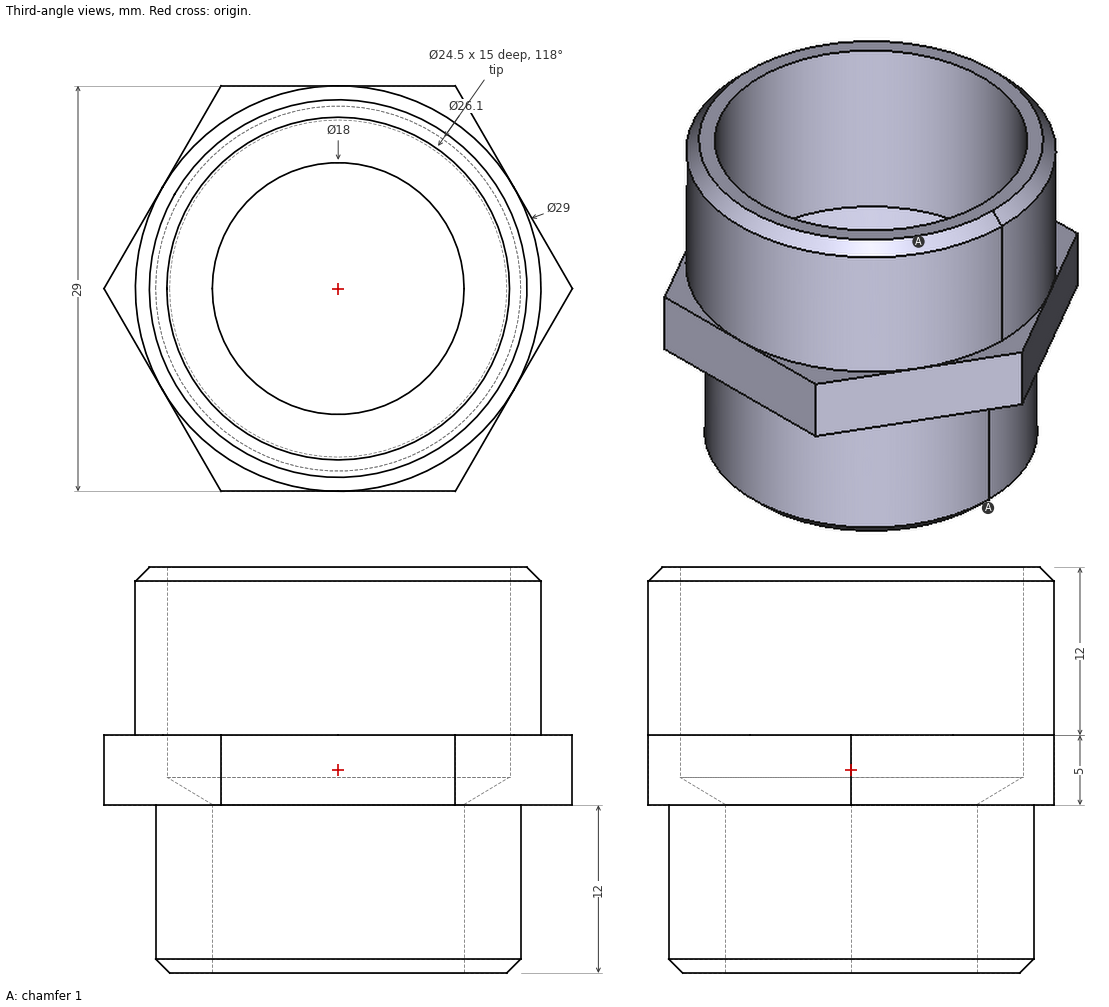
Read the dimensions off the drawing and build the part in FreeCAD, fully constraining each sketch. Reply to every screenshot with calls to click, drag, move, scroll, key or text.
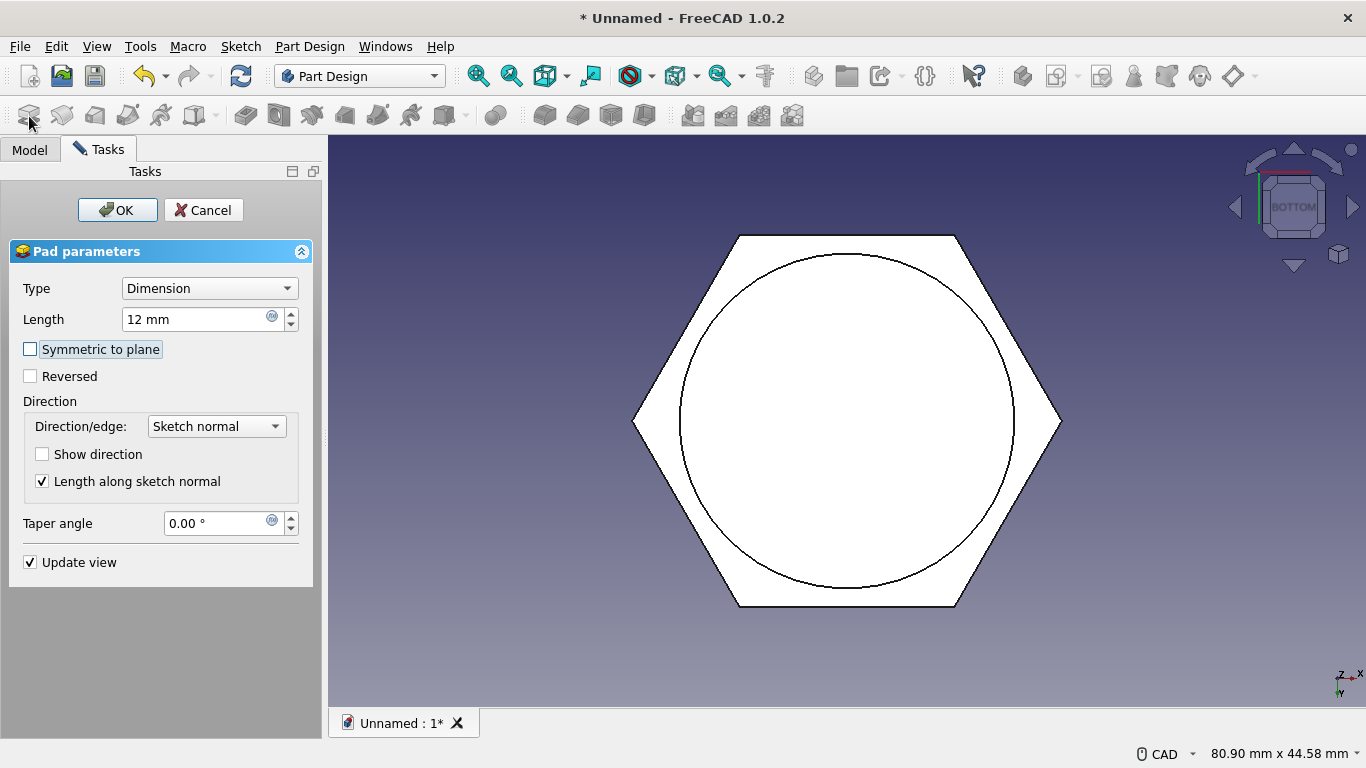
click(118, 210)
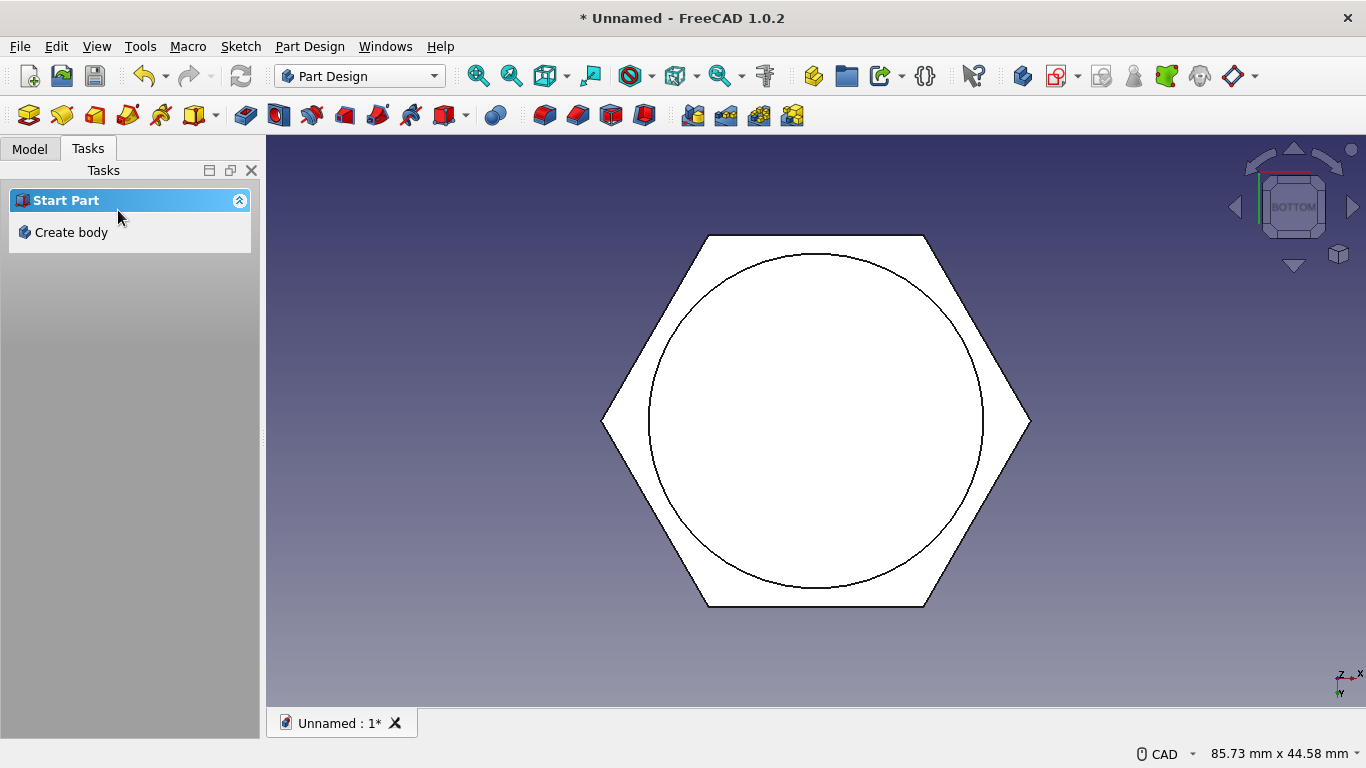
click(816, 420)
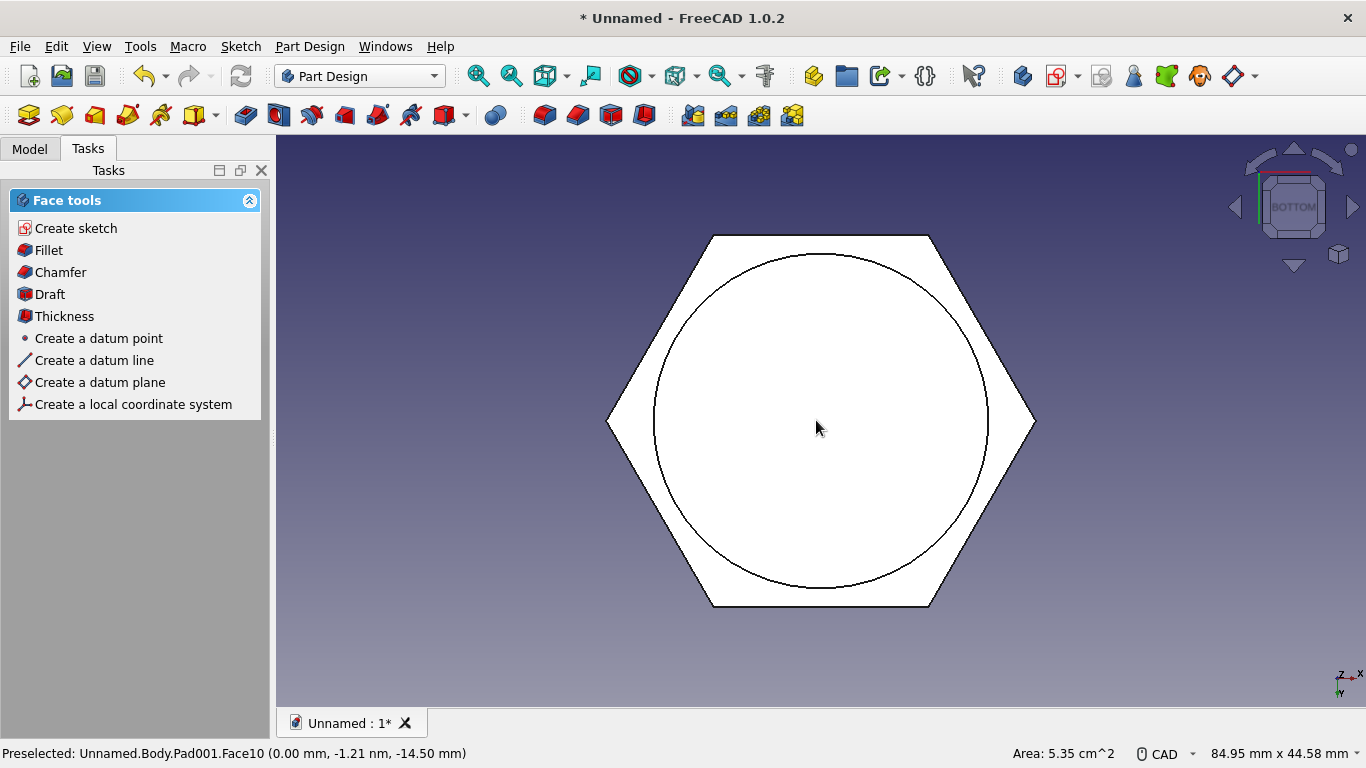
click(1056, 76)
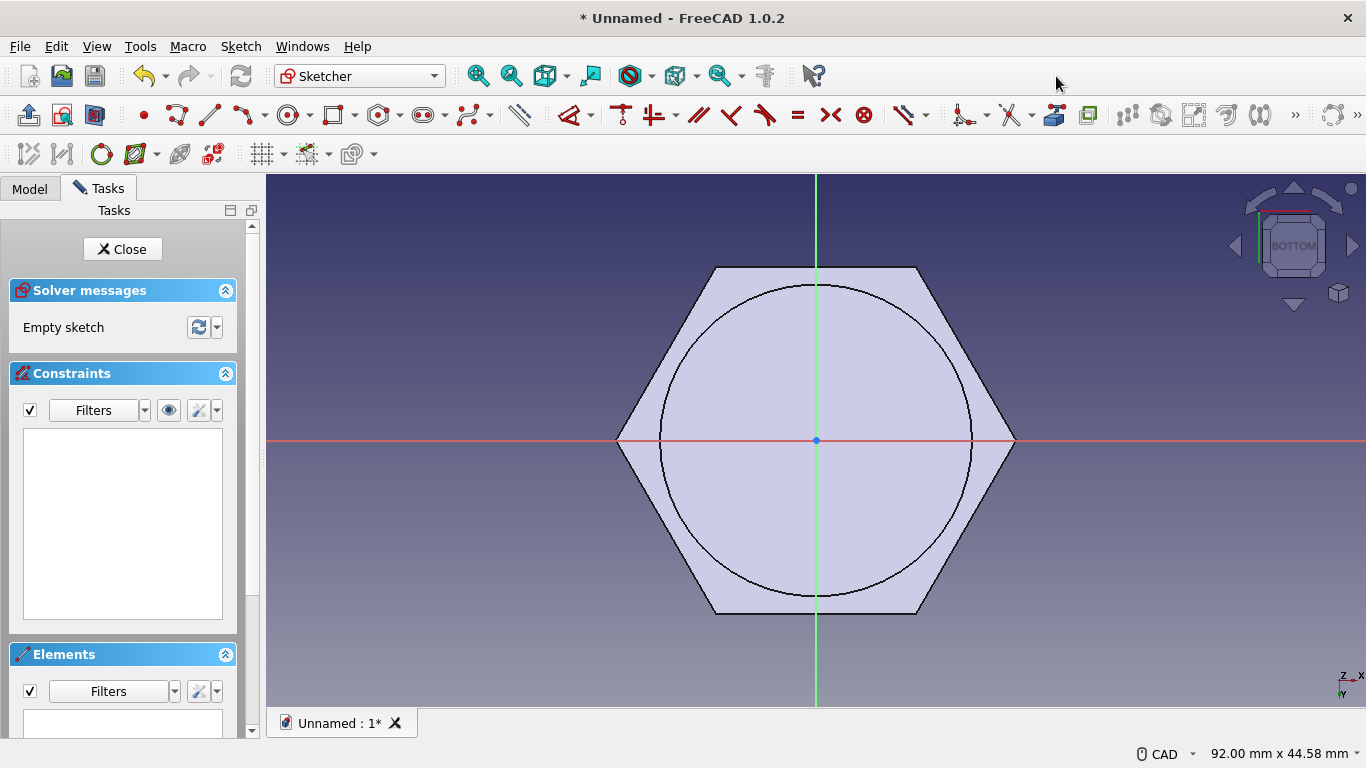
scroll(955, 441, up, 2)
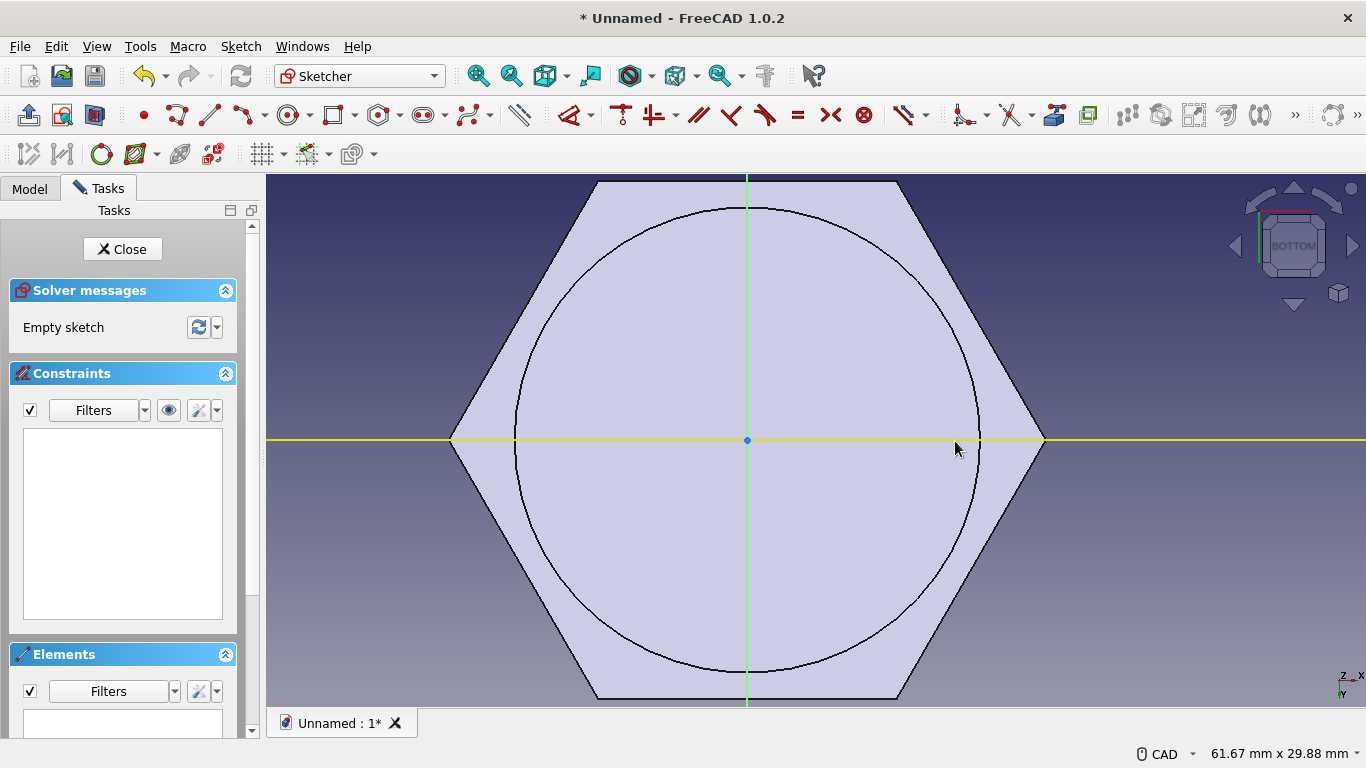
click(288, 116)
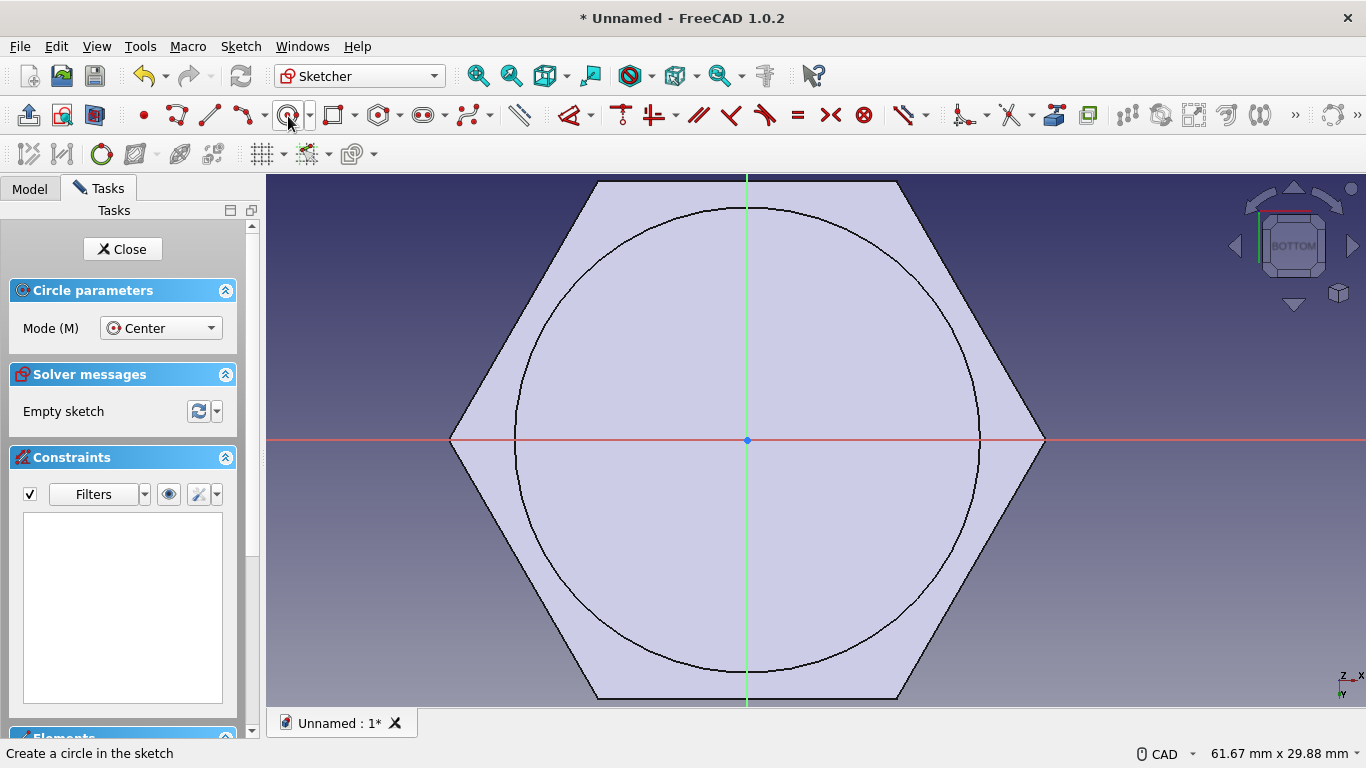
click(747, 440)
move(861, 326)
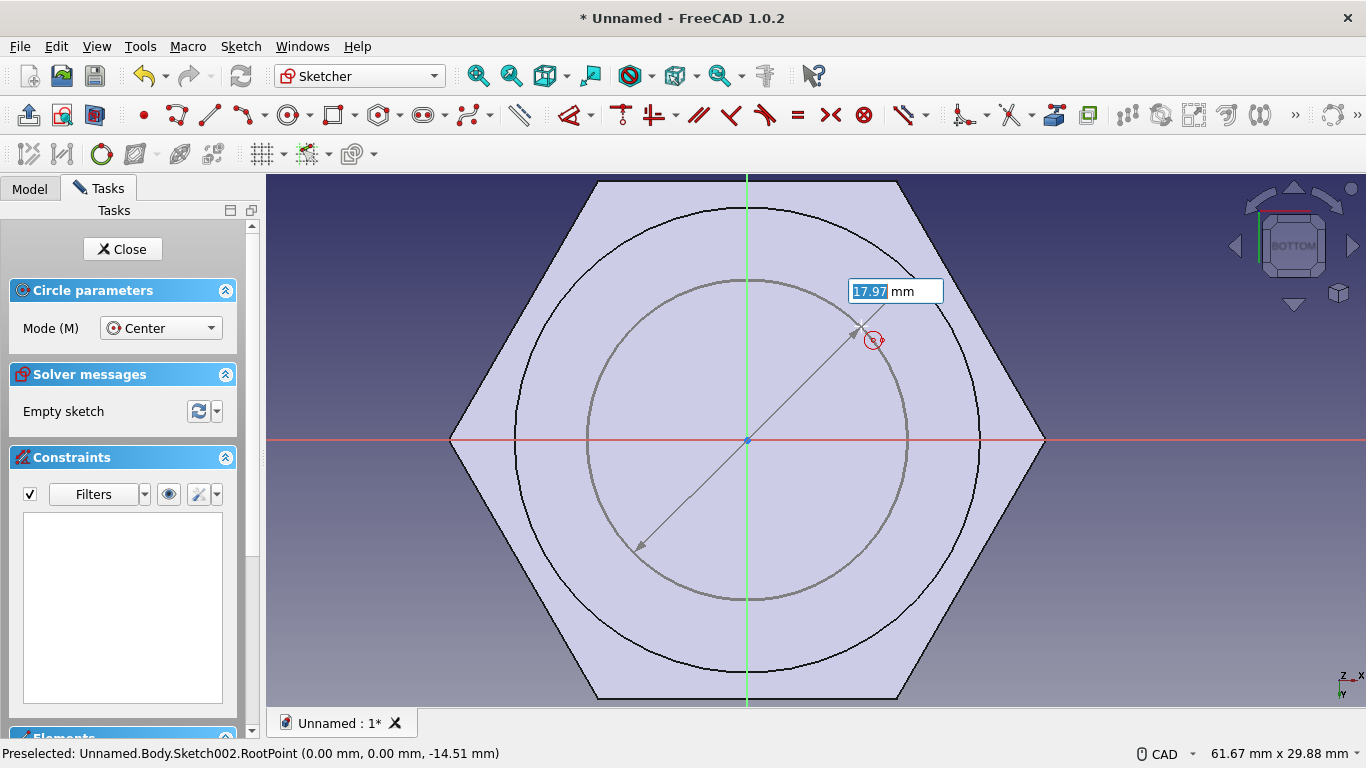
text(18)
key(Return)
key(Escape)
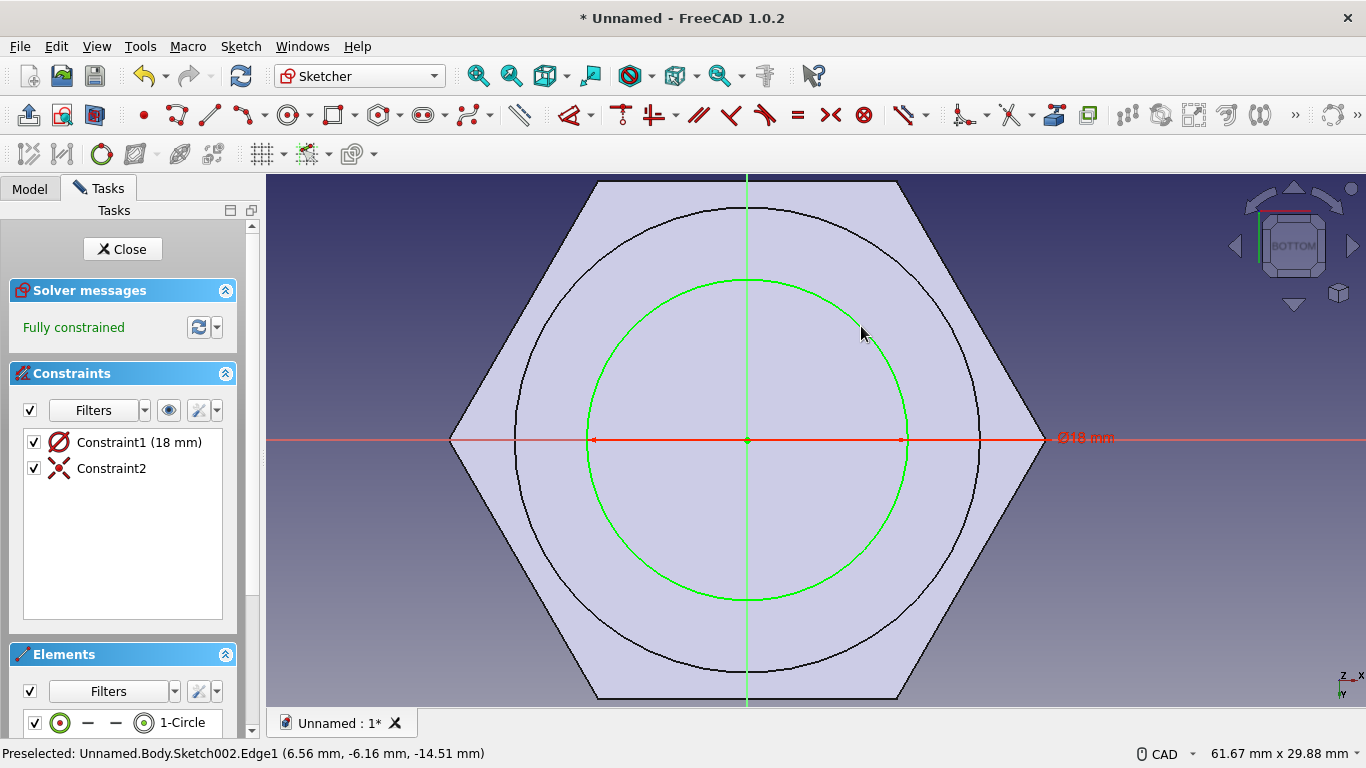
click(123, 249)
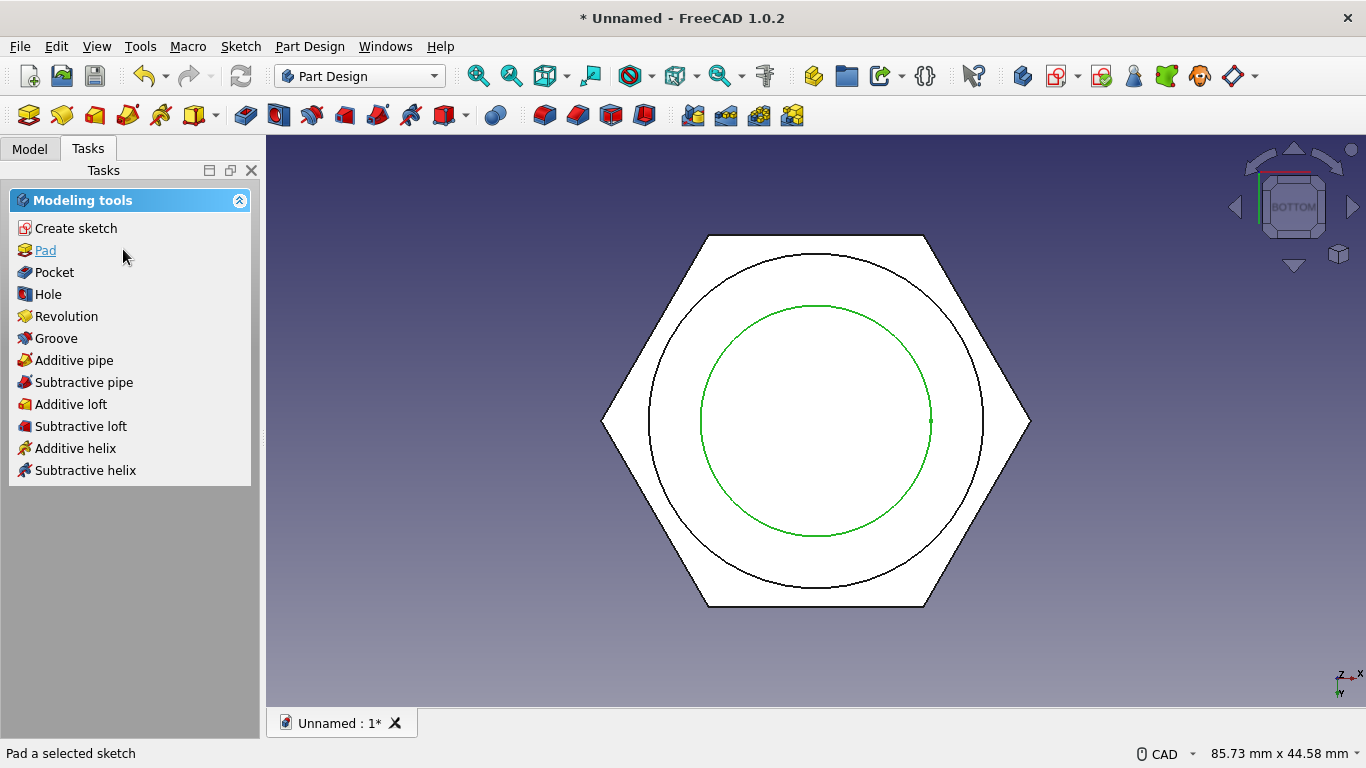
click(246, 116)